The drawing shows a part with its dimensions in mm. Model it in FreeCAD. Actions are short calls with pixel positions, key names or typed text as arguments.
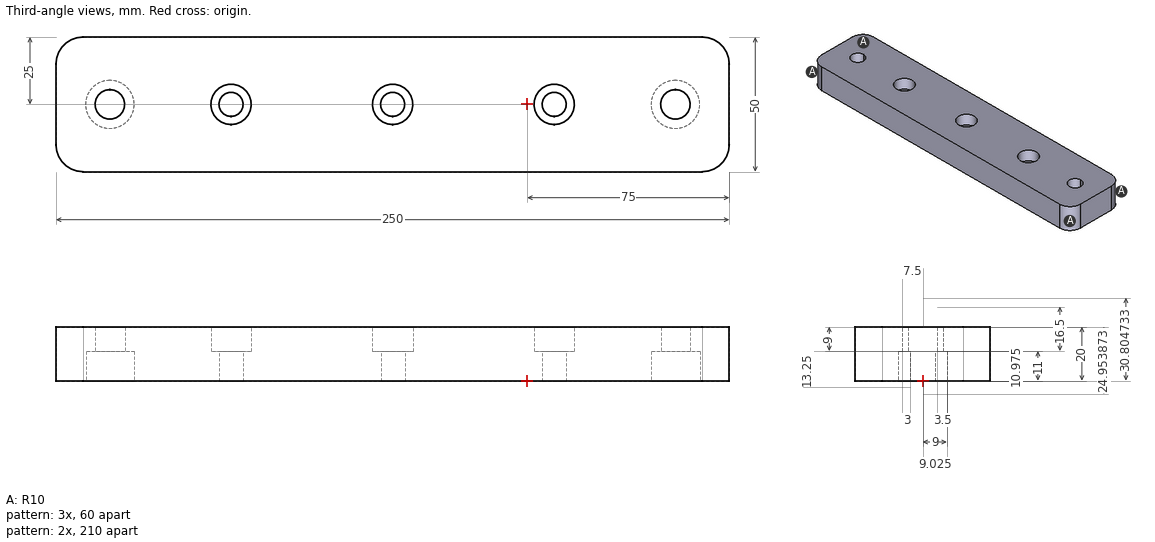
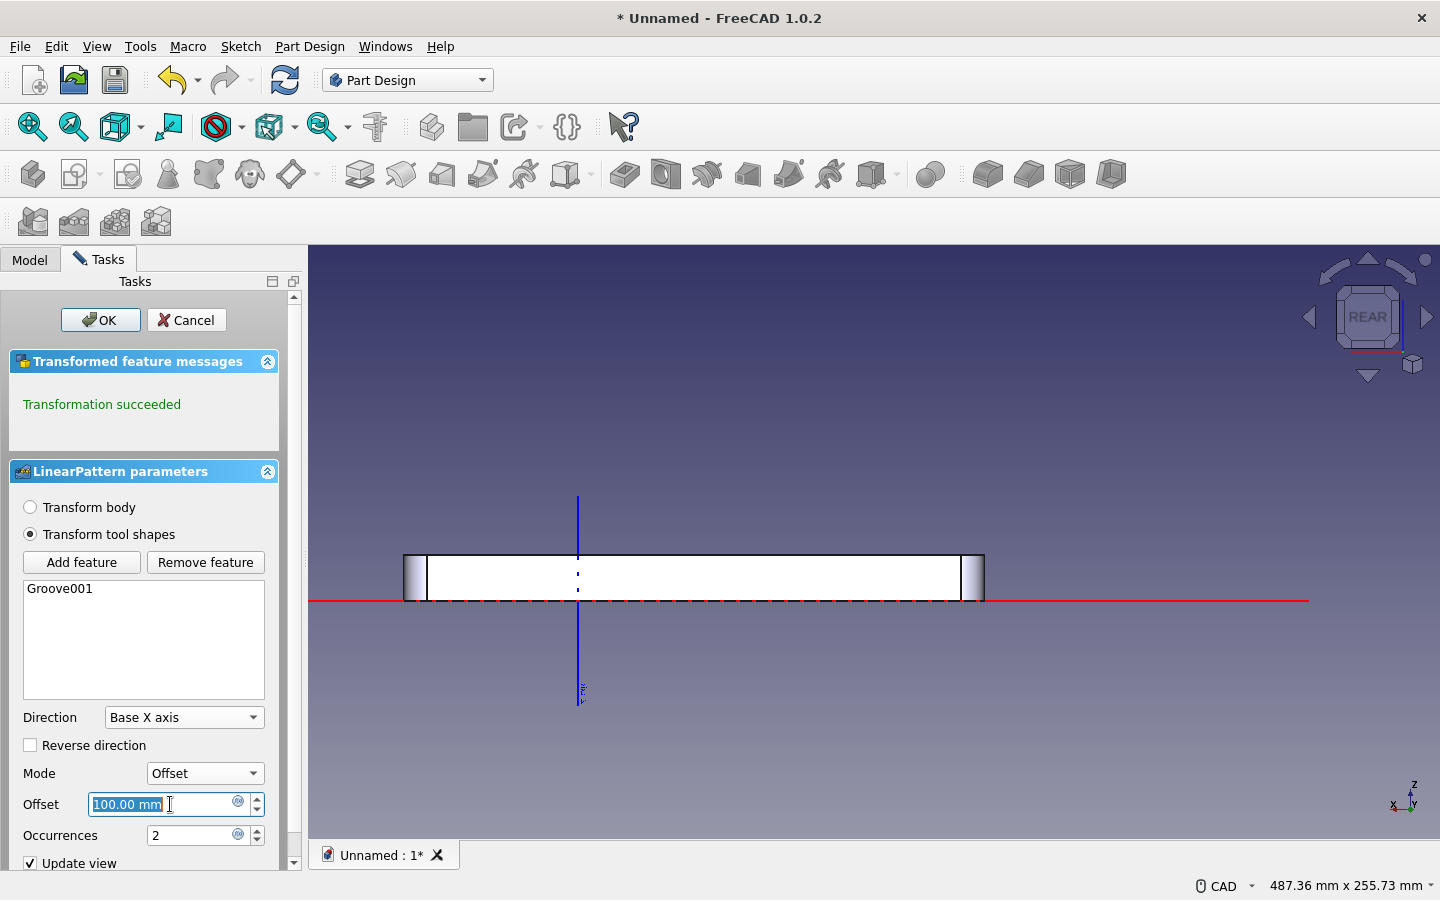
text(210)
key(Tab)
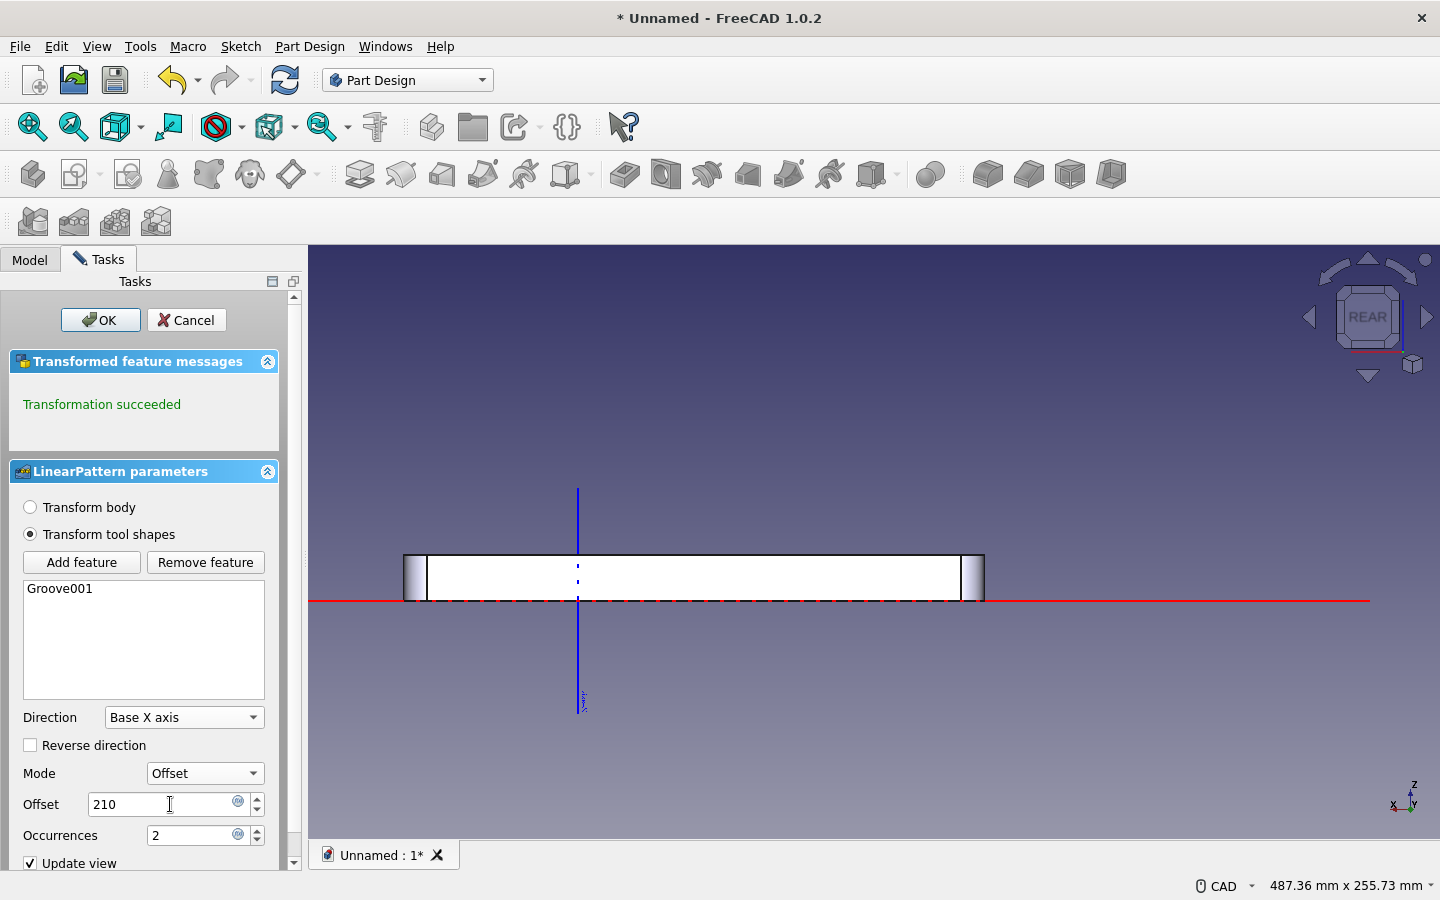
triple_click(199, 836)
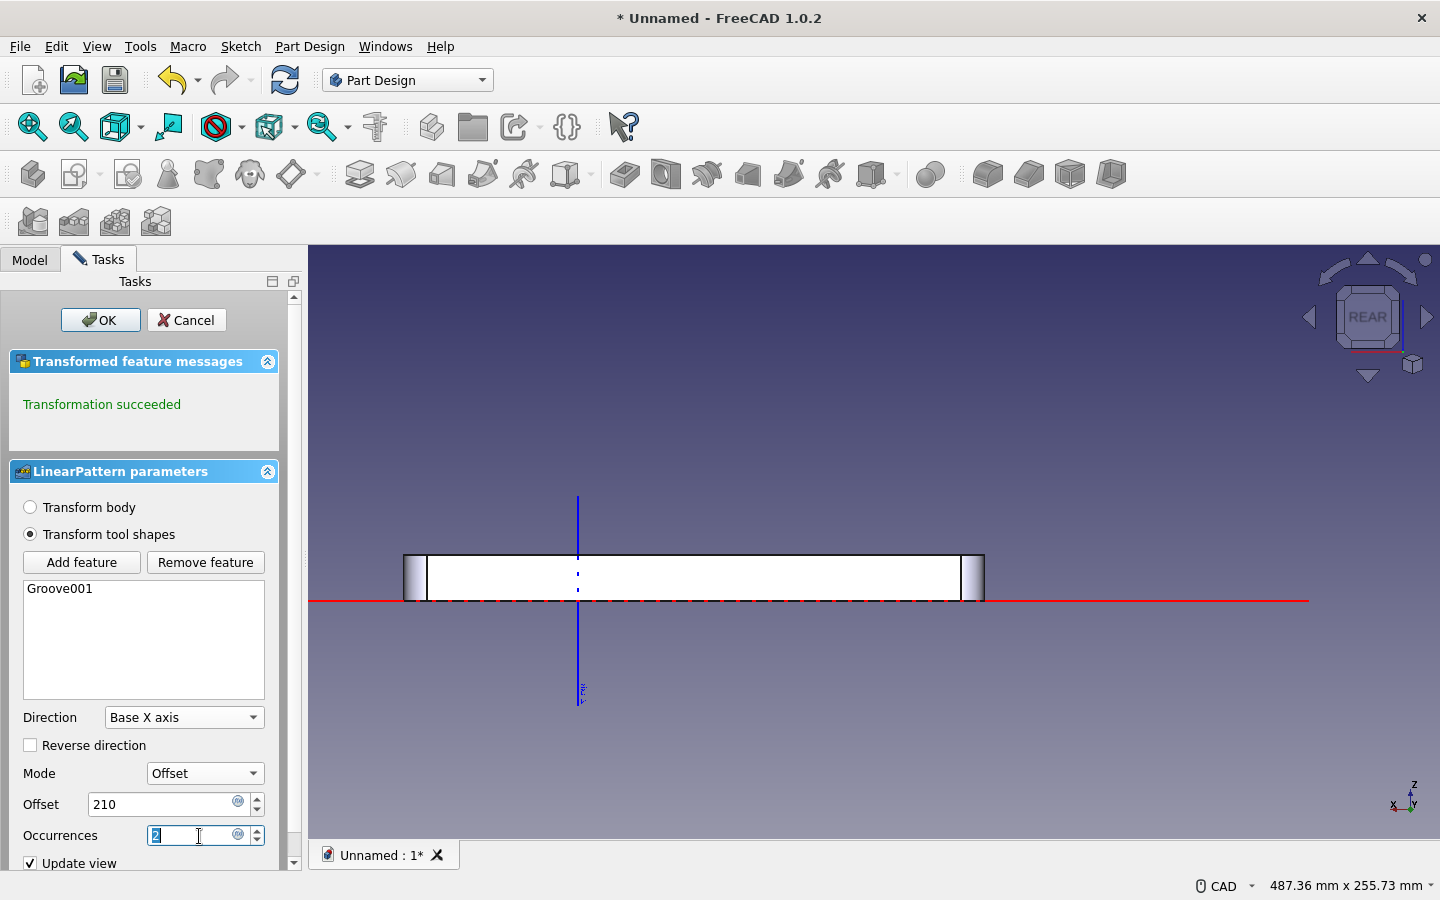
text(2)
key(Tab)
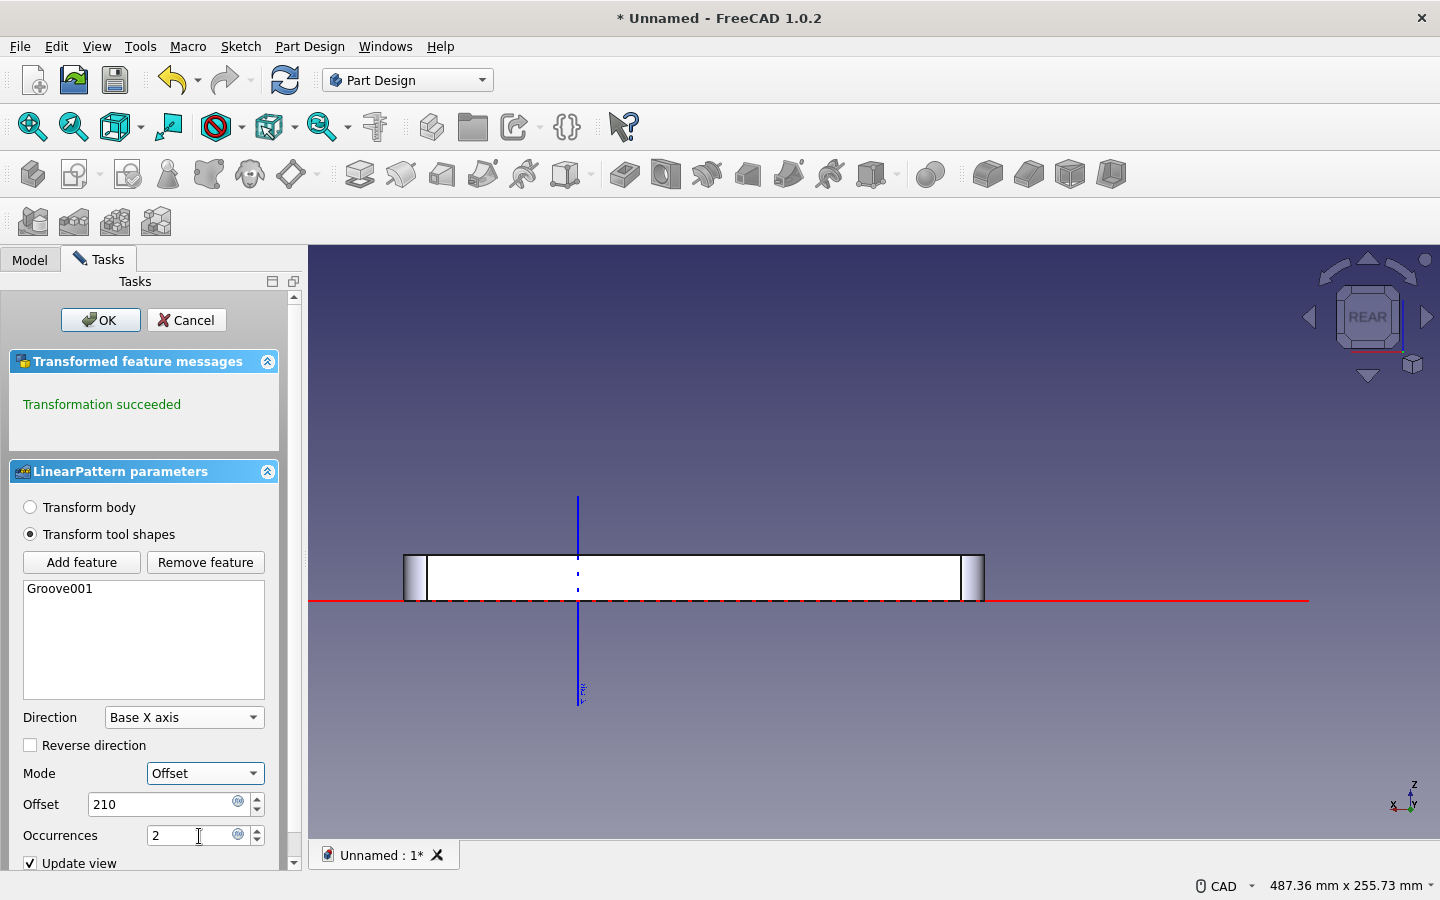
click(31, 745)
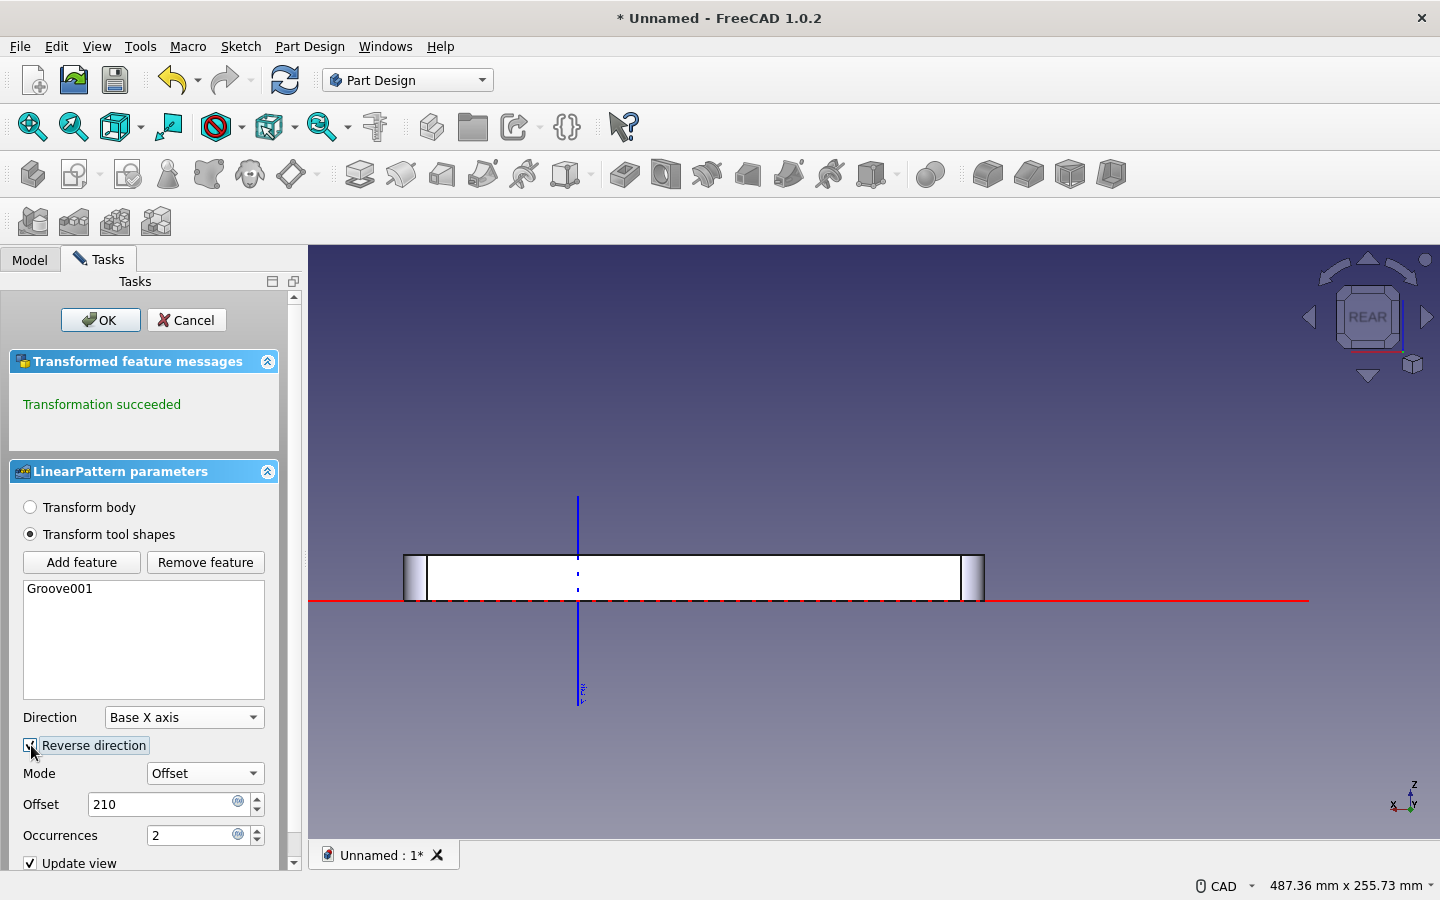
click(101, 320)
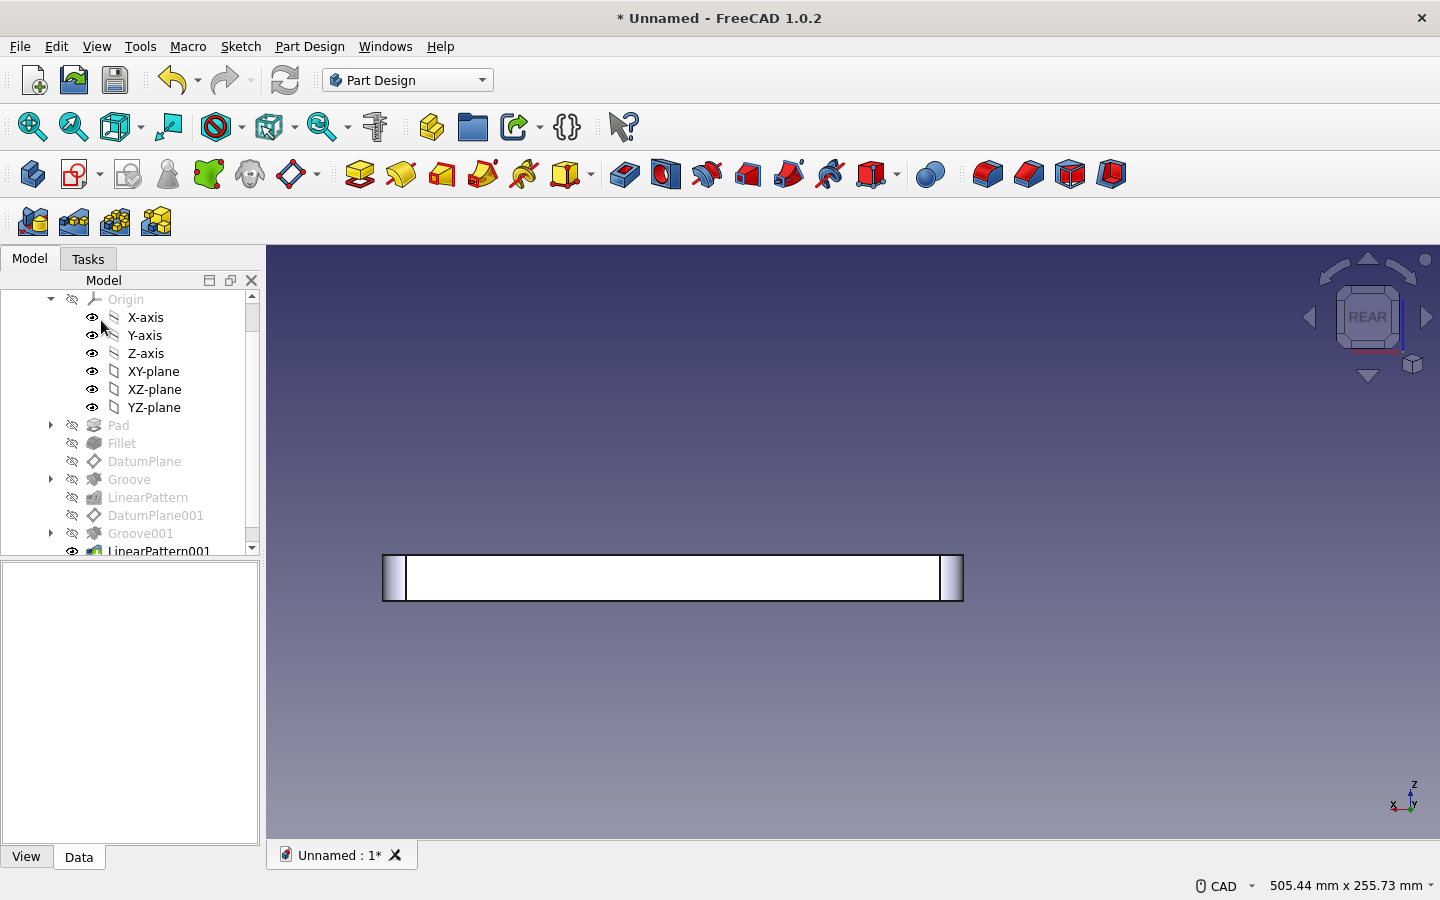
key(0)